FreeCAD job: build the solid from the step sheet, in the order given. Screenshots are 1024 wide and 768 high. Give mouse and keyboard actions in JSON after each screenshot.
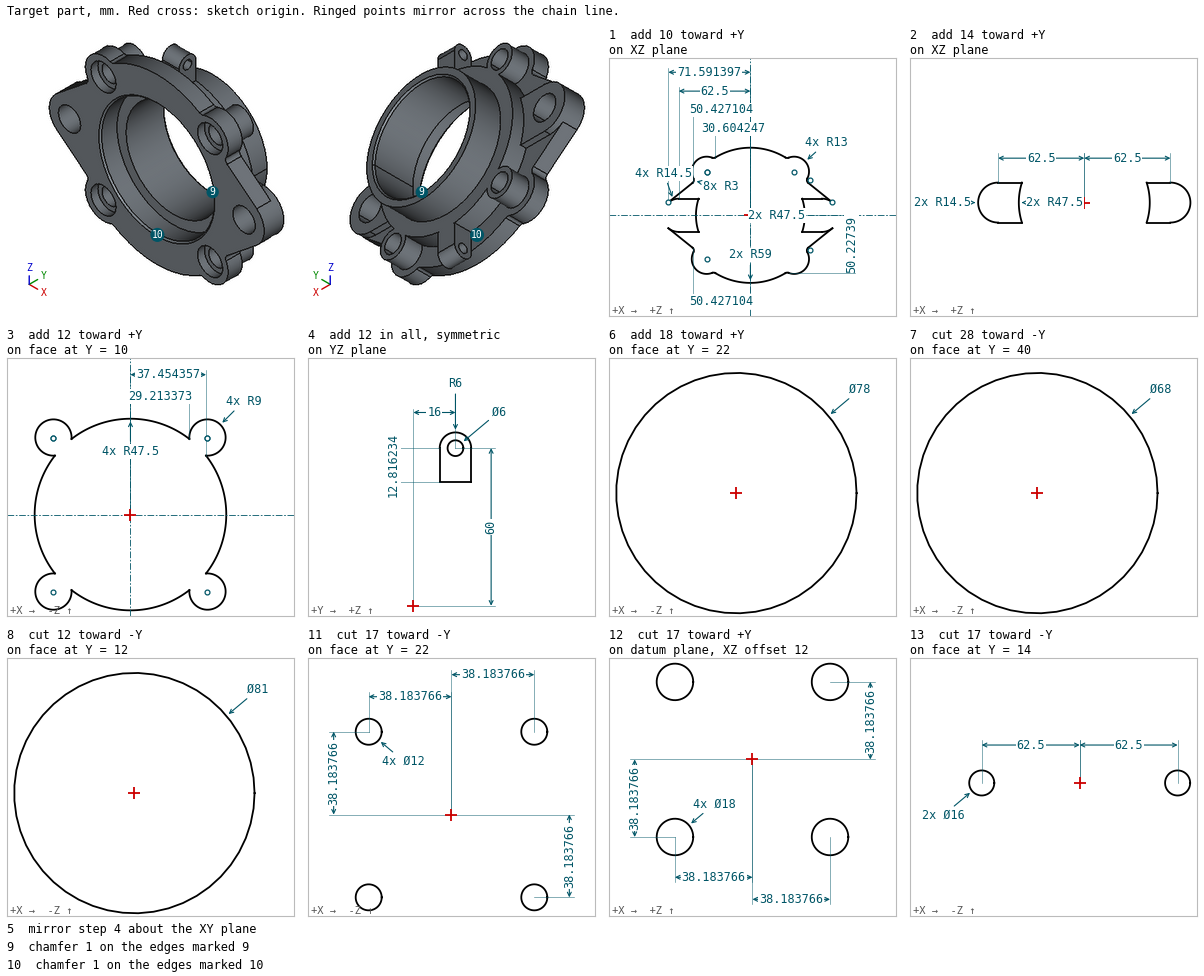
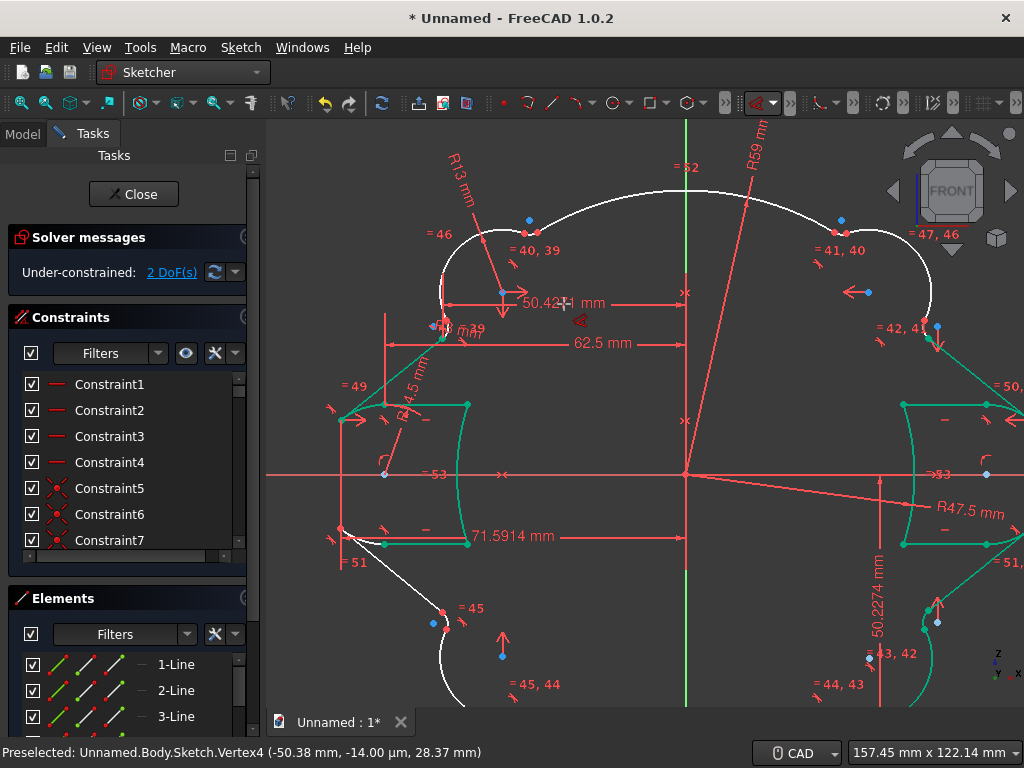
{"action": "left_click", "coordinate": [442, 612]}
{"action": "left_click", "coordinate": [564, 646]}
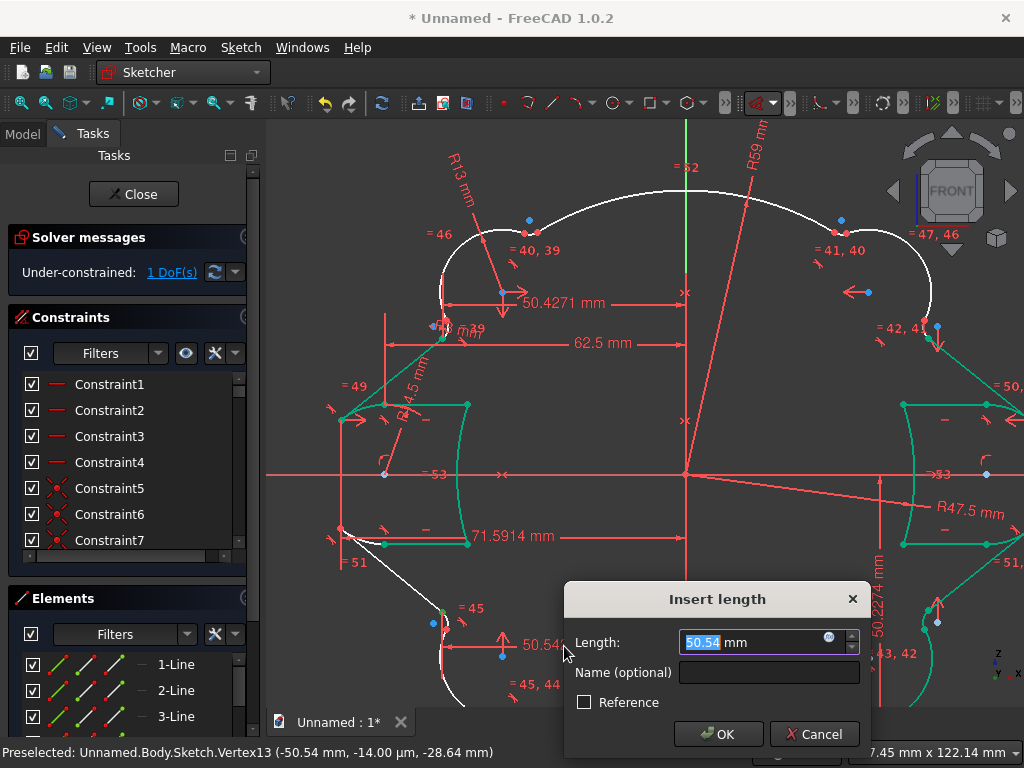
{"action": "type", "text": "50.427104"}
{"action": "key", "text": "Return"}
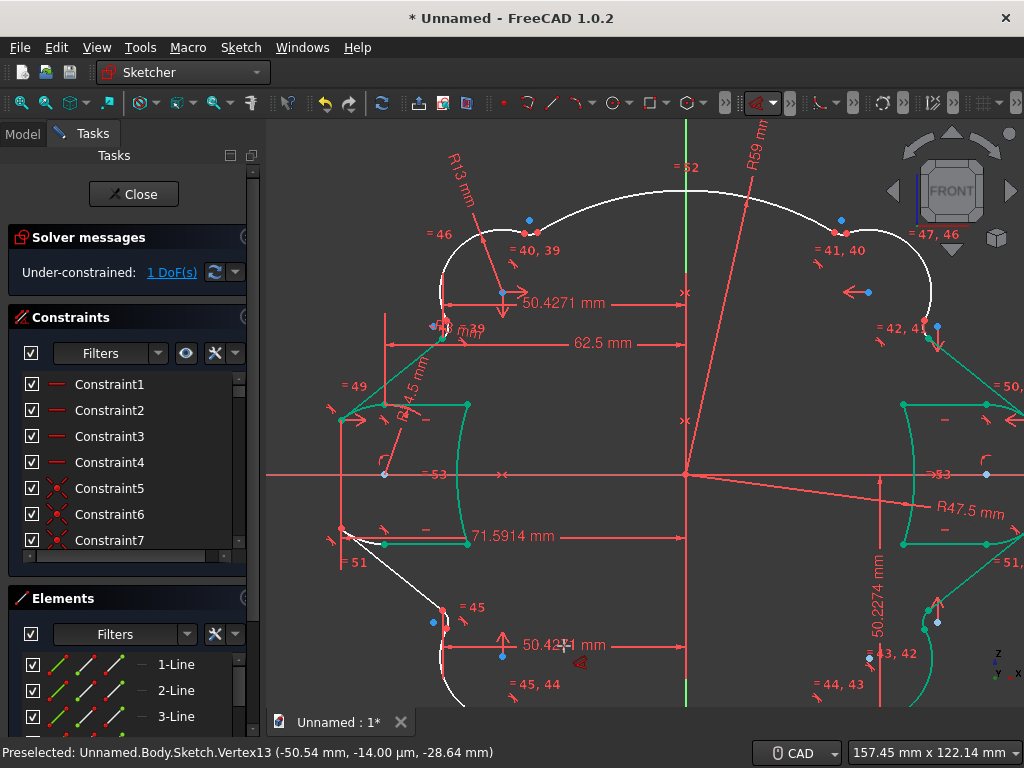
{"action": "left_click", "coordinate": [537, 232]}
{"action": "left_click", "coordinate": [560, 198]}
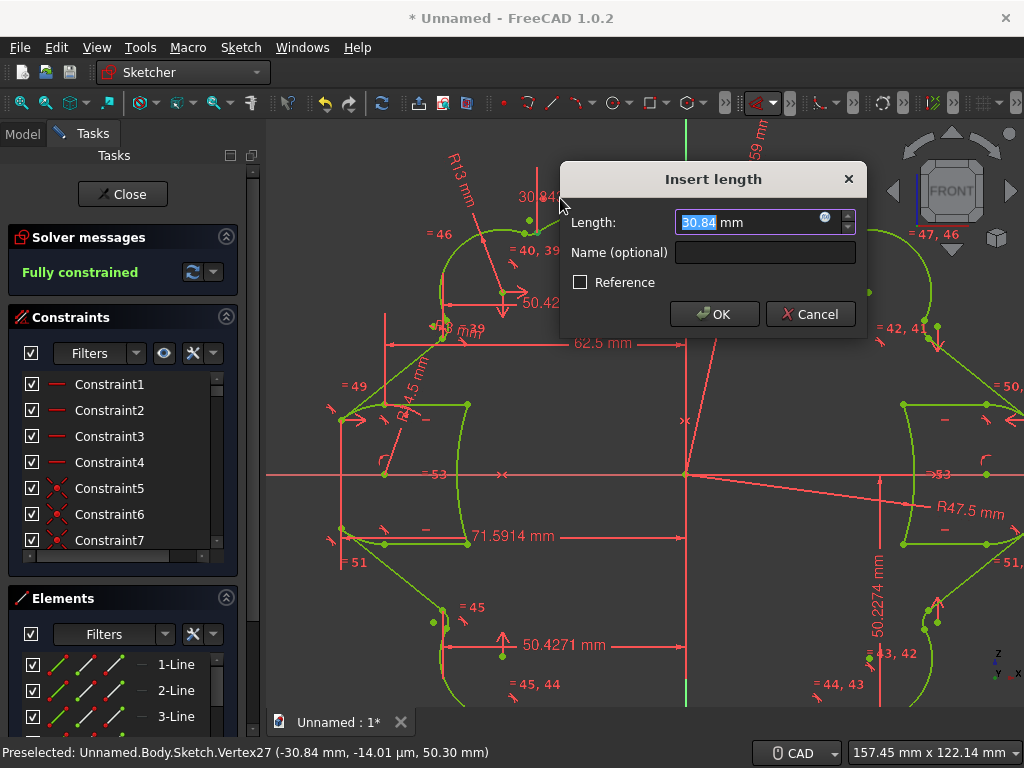
{"action": "type", "text": "30.604247"}
{"action": "key", "text": "Return"}
{"action": "key", "text": "Escape"}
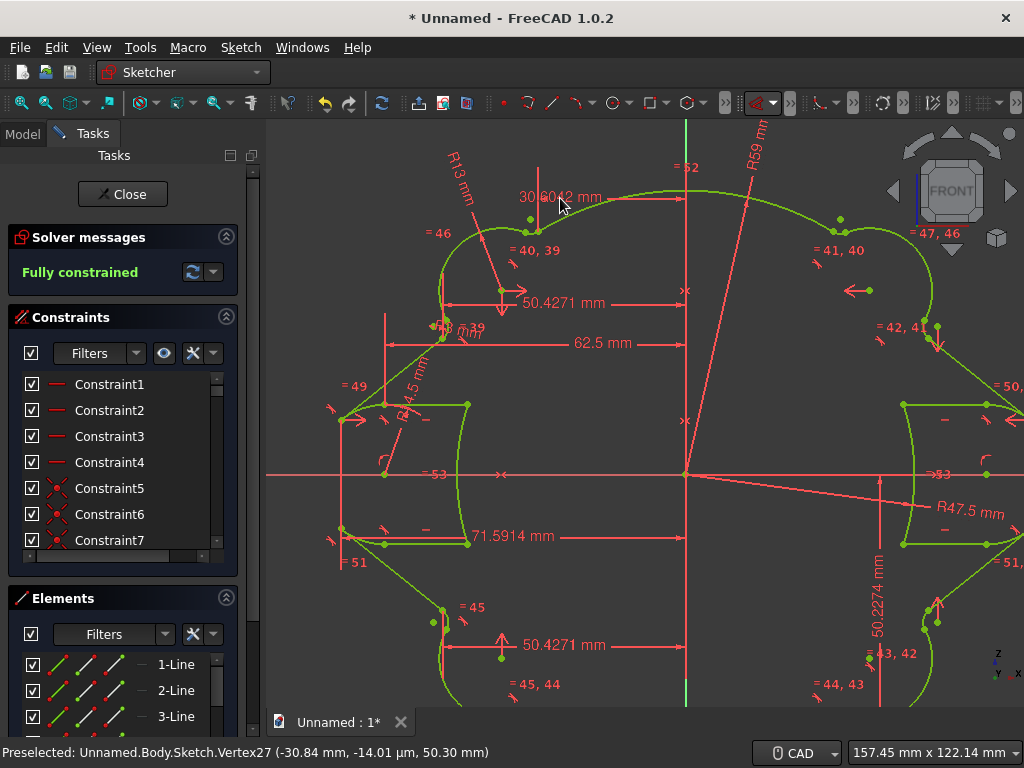
{"action": "left_click", "coordinate": [123, 194]}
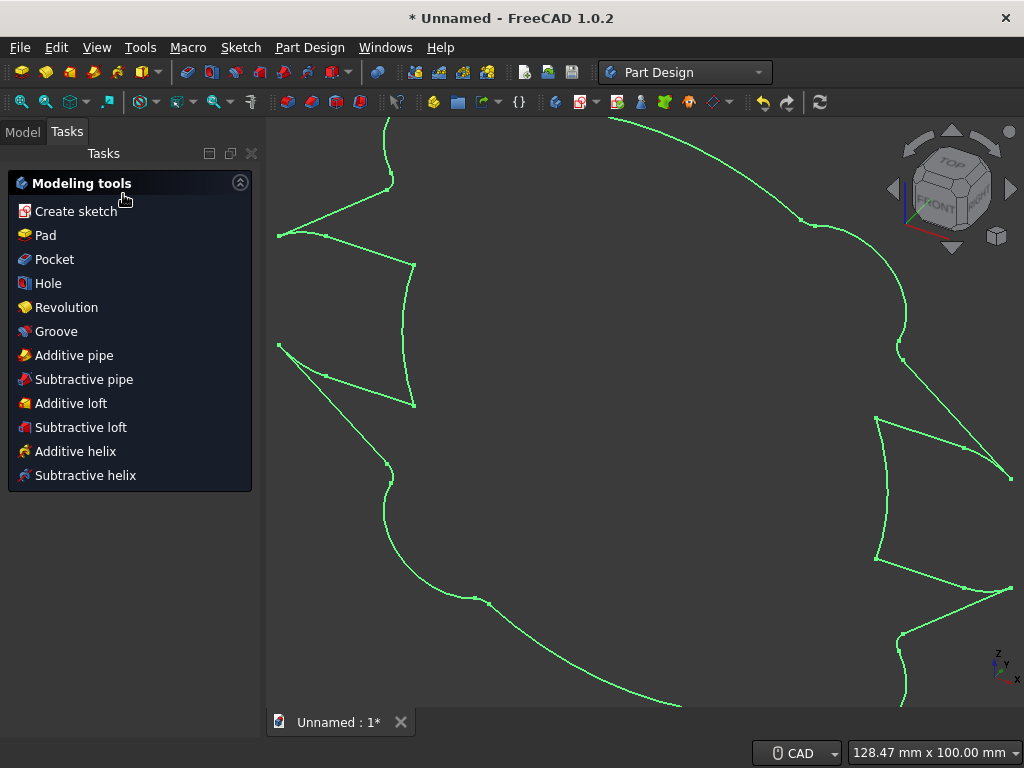
{"action": "left_click", "coordinate": [22, 72]}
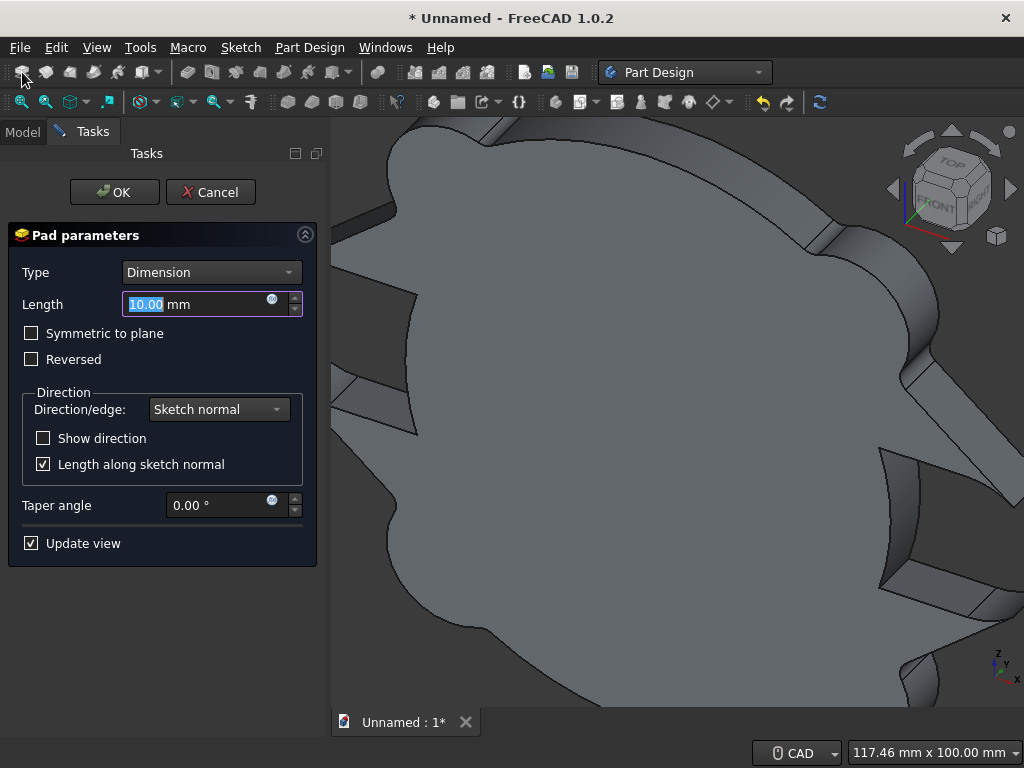
{"action": "type", "text": "10"}
{"action": "key", "text": "Tab"}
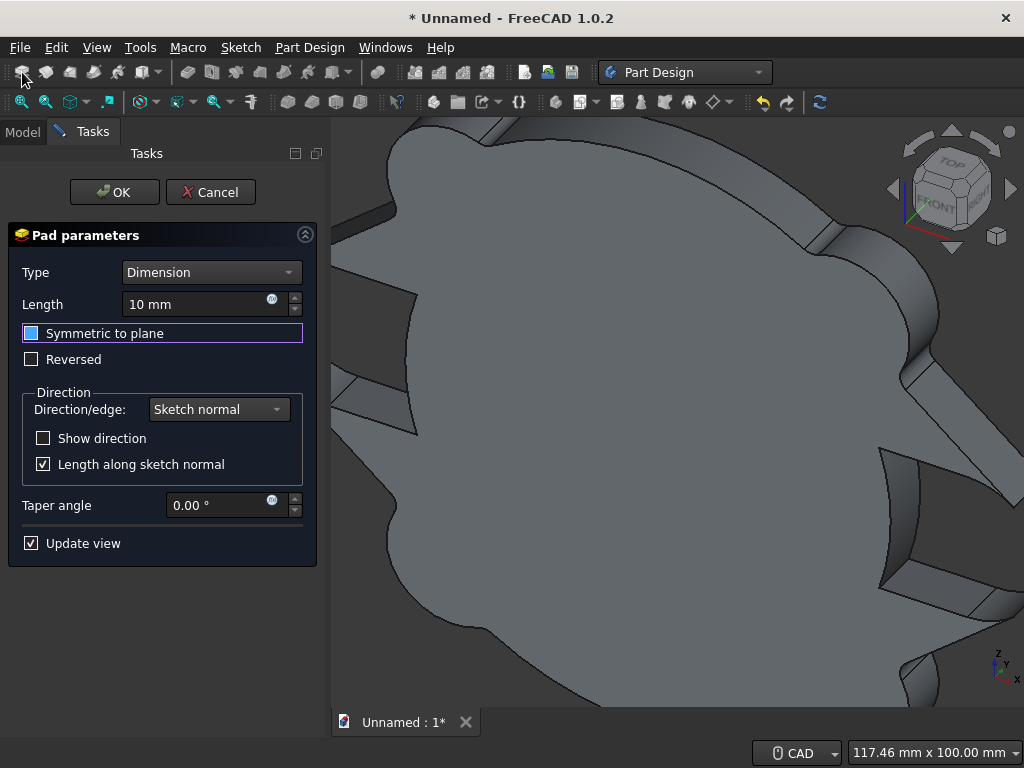
{"action": "left_click", "coordinate": [30, 359]}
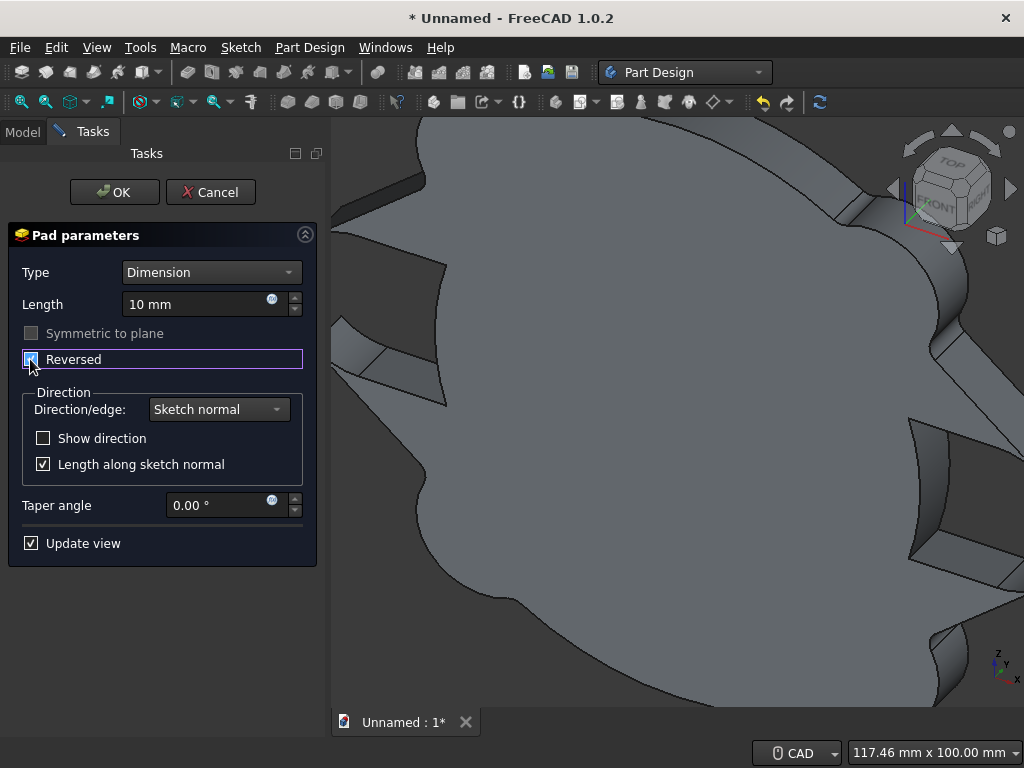
{"action": "left_click", "coordinate": [115, 192]}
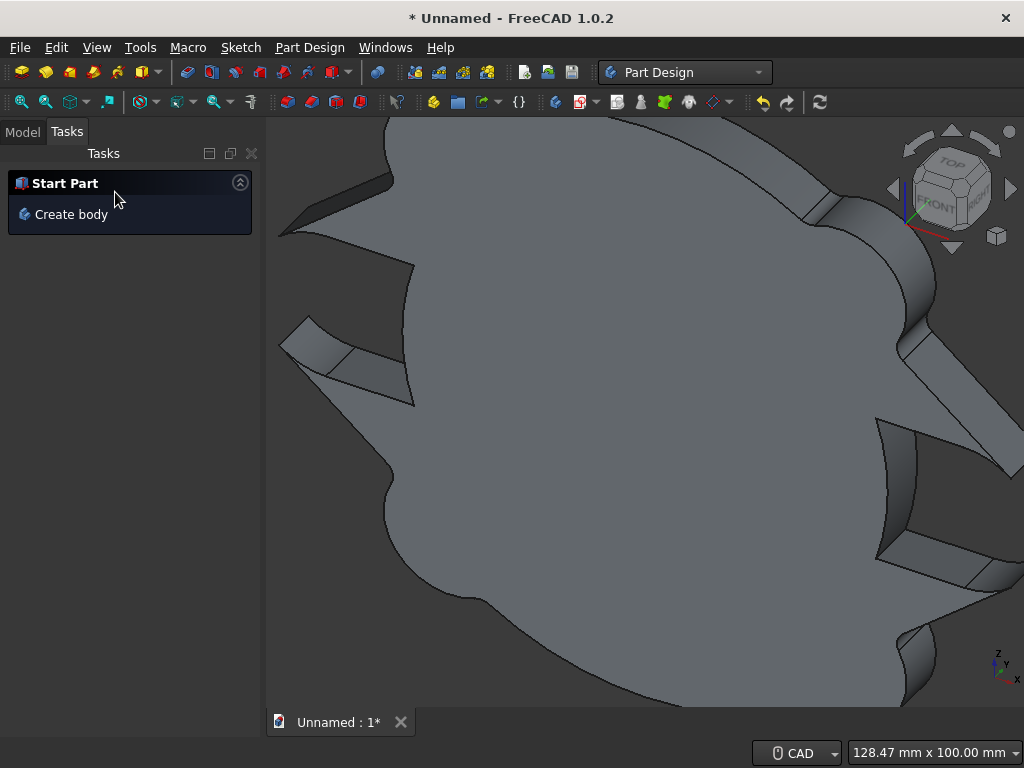
{"action": "key", "text": "v f"}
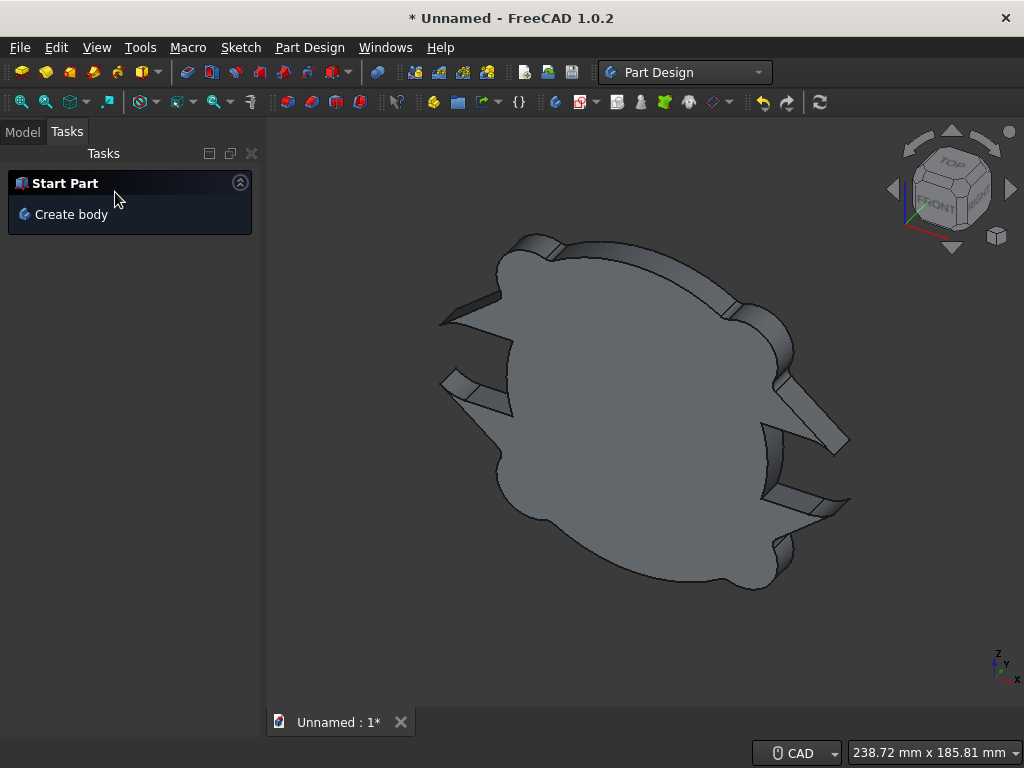
{"action": "left_click", "coordinate": [580, 102]}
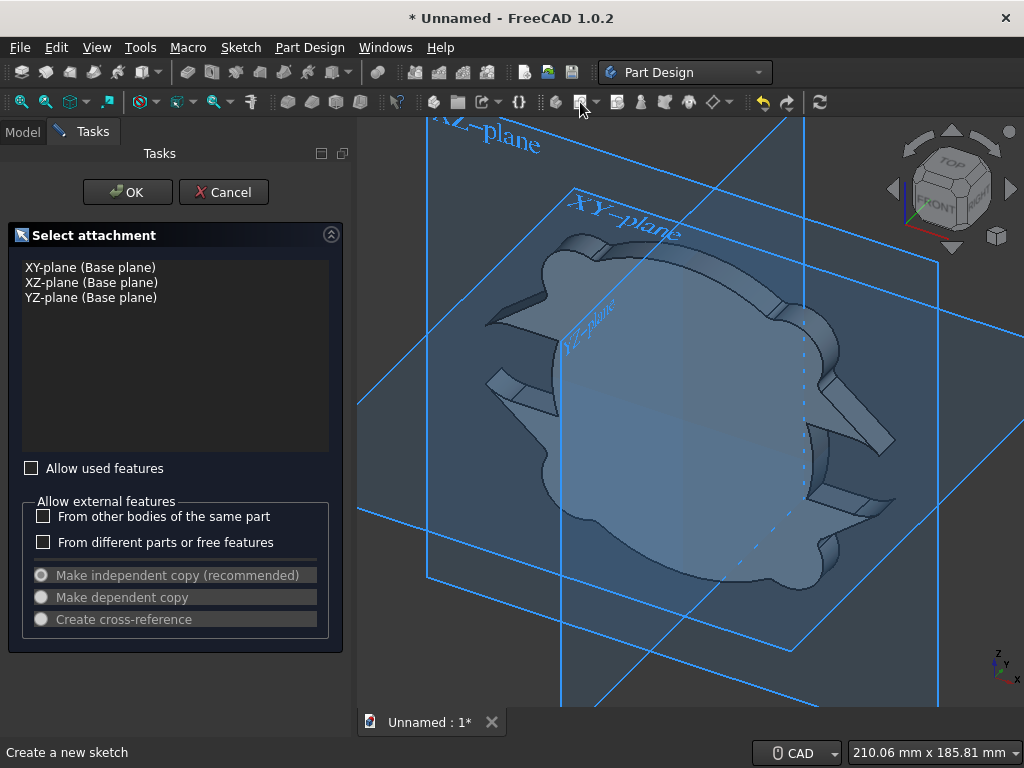
{"action": "left_click", "coordinate": [82, 282]}